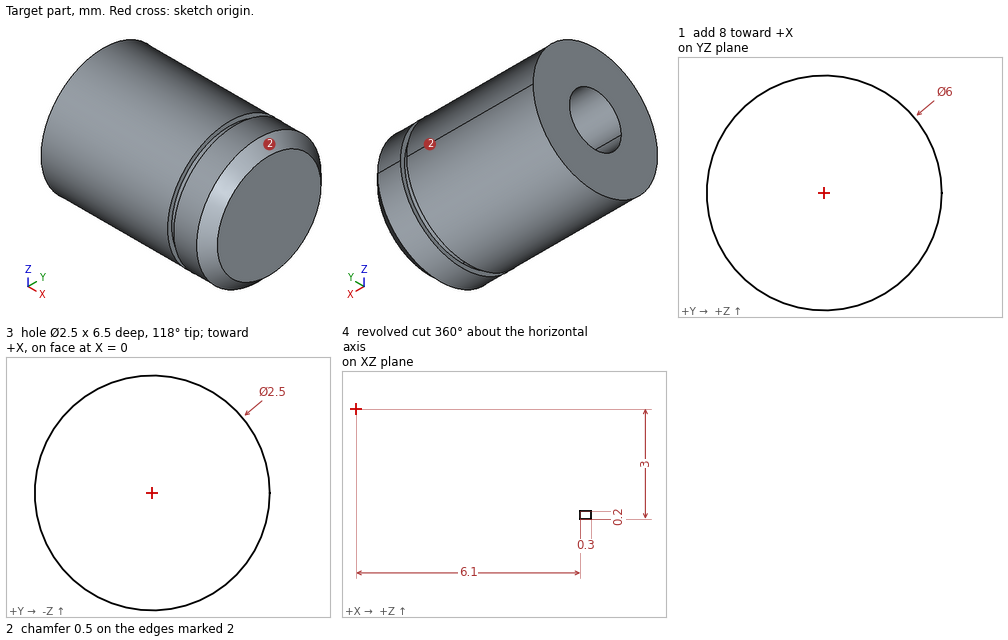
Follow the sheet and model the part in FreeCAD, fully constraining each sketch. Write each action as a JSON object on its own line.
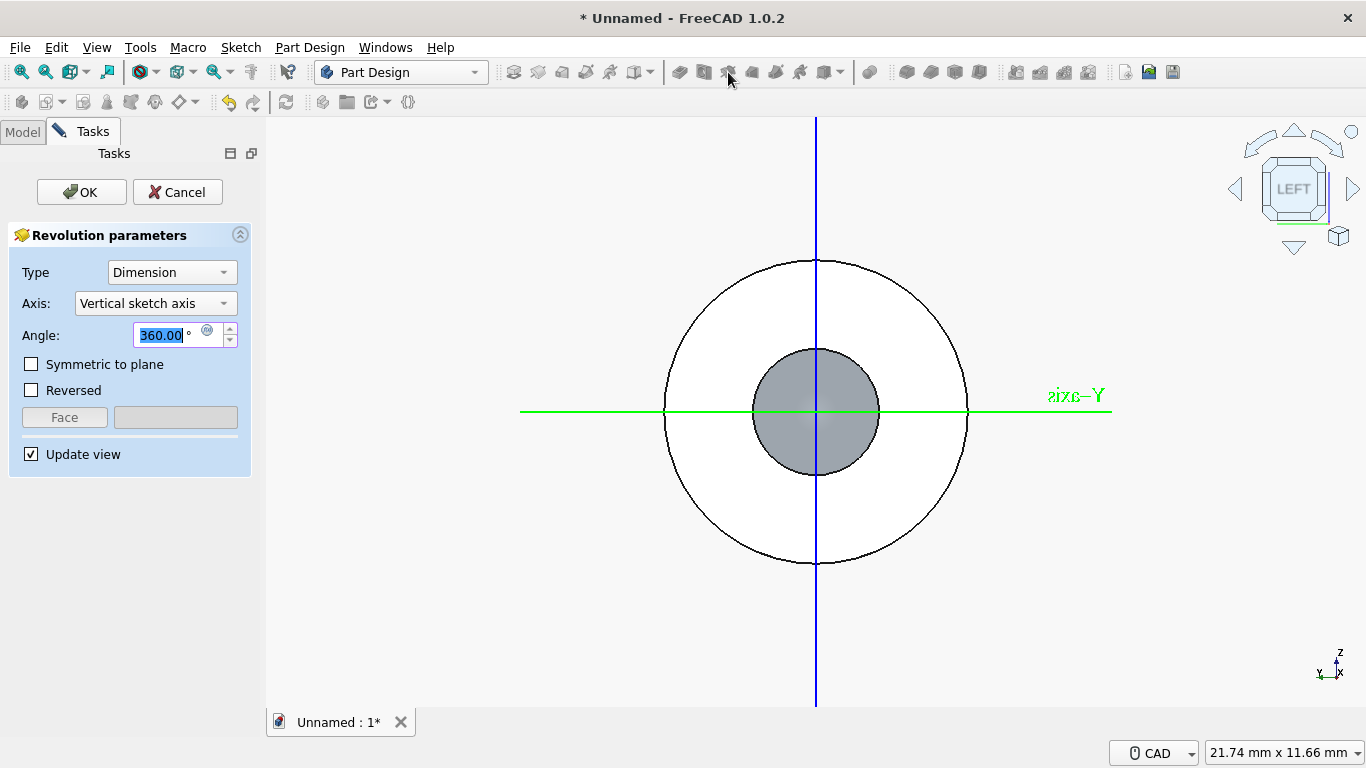
{"action": "left_click", "coordinate": [156, 304]}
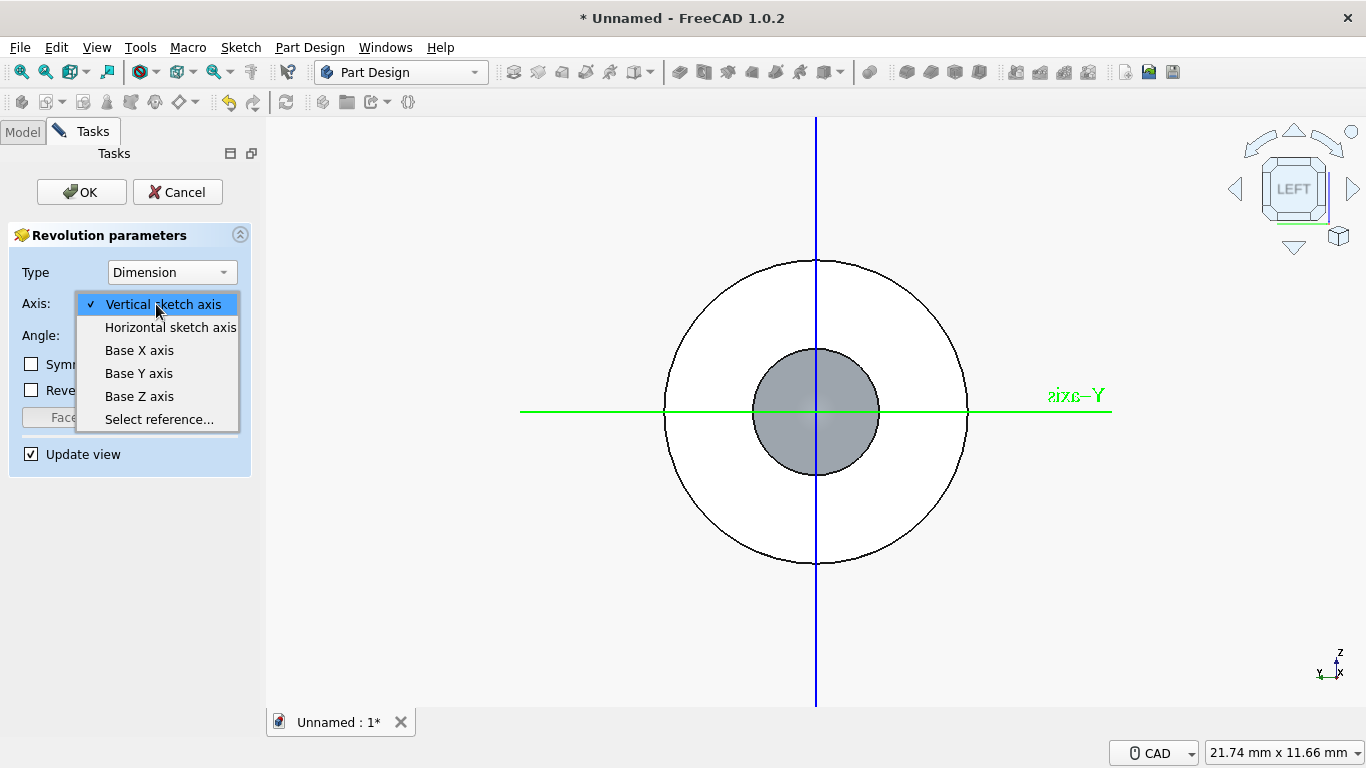
{"action": "left_click", "coordinate": [156, 328]}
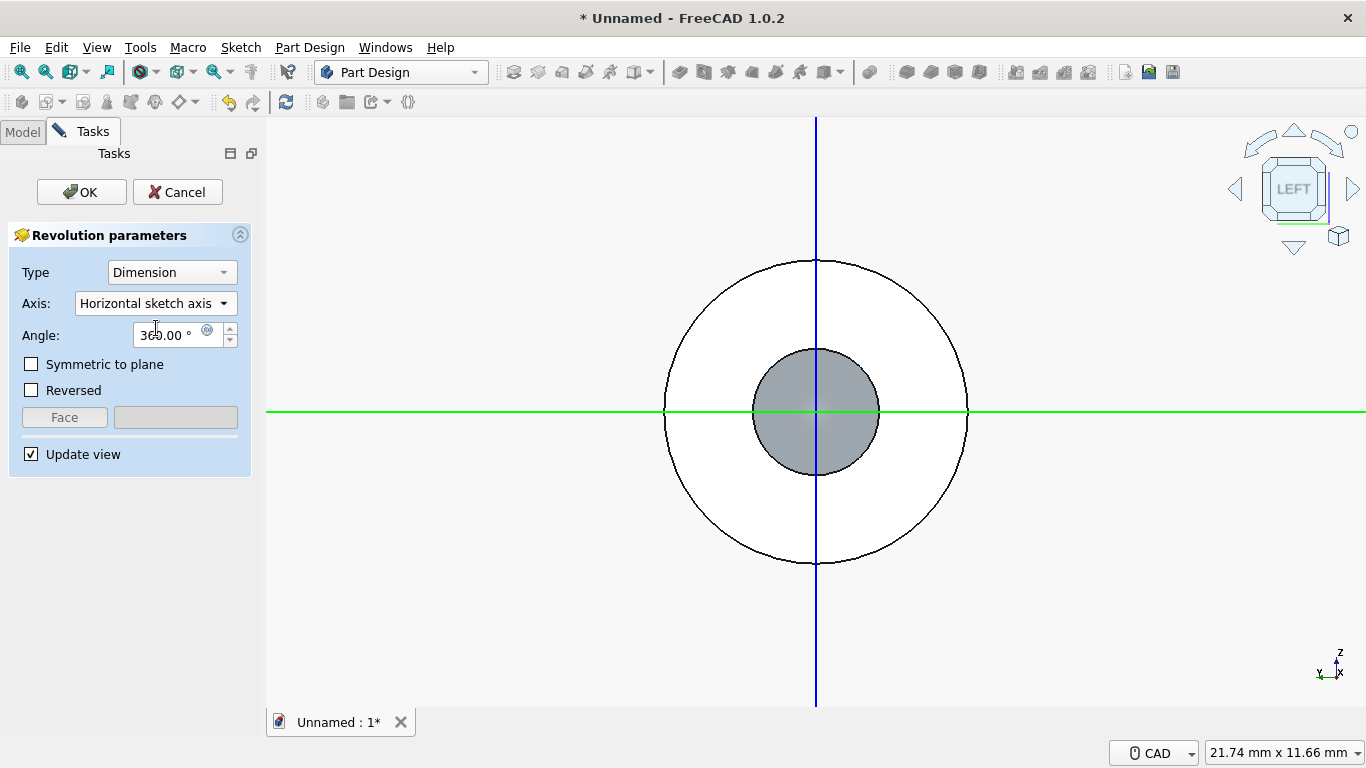
{"action": "left_click", "coordinate": [82, 192]}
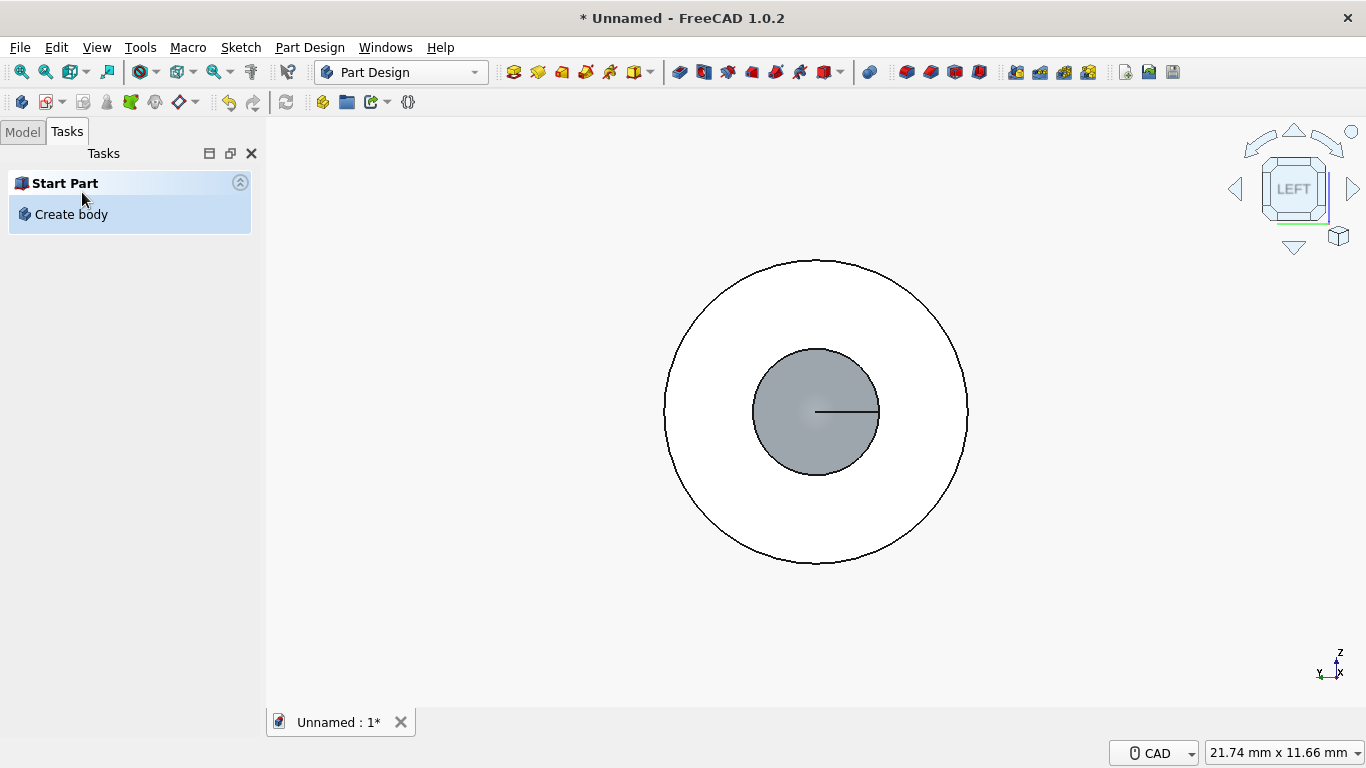
{"action": "key", "text": "0"}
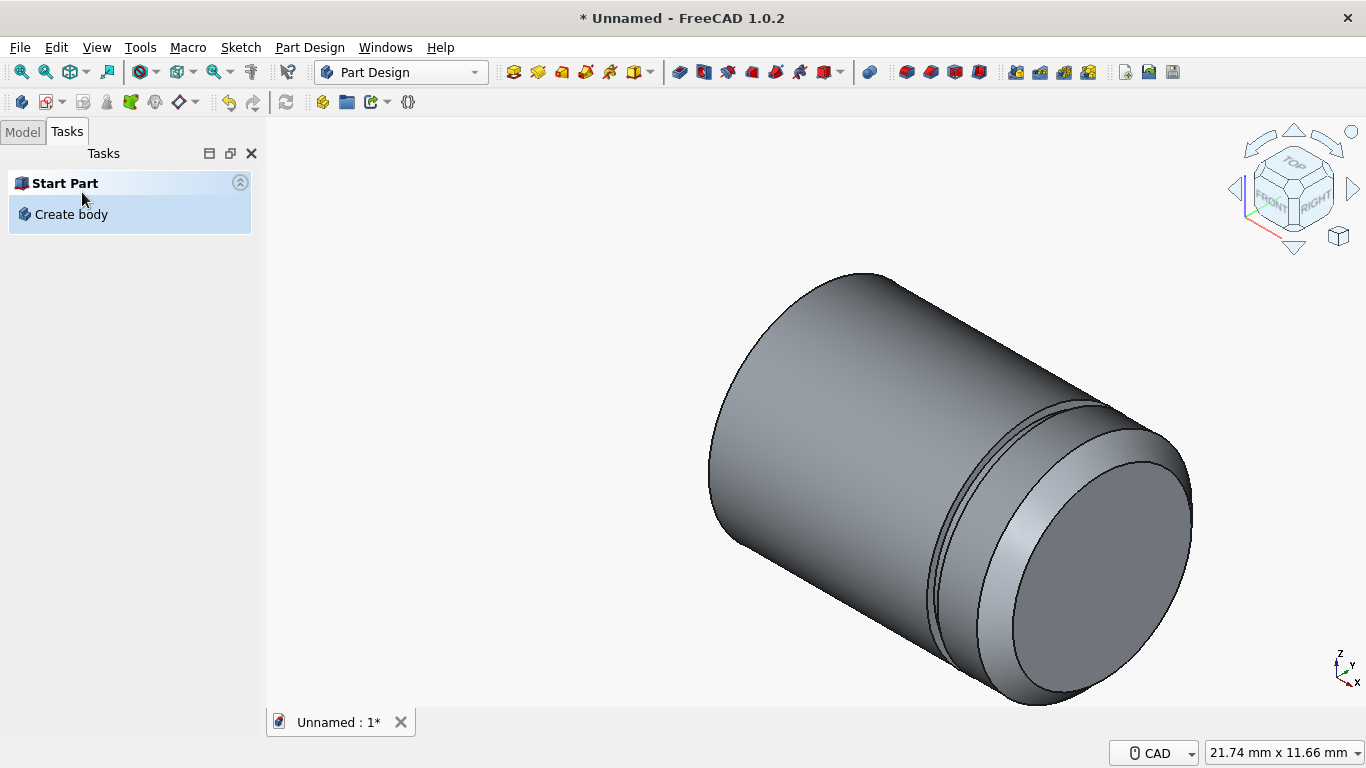
{"action": "key", "text": "v f"}